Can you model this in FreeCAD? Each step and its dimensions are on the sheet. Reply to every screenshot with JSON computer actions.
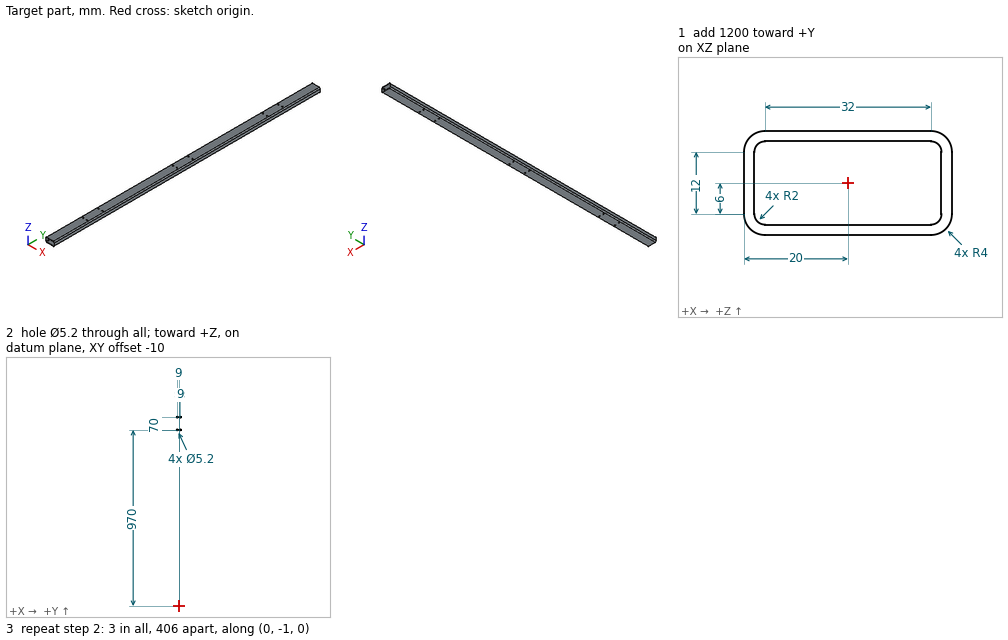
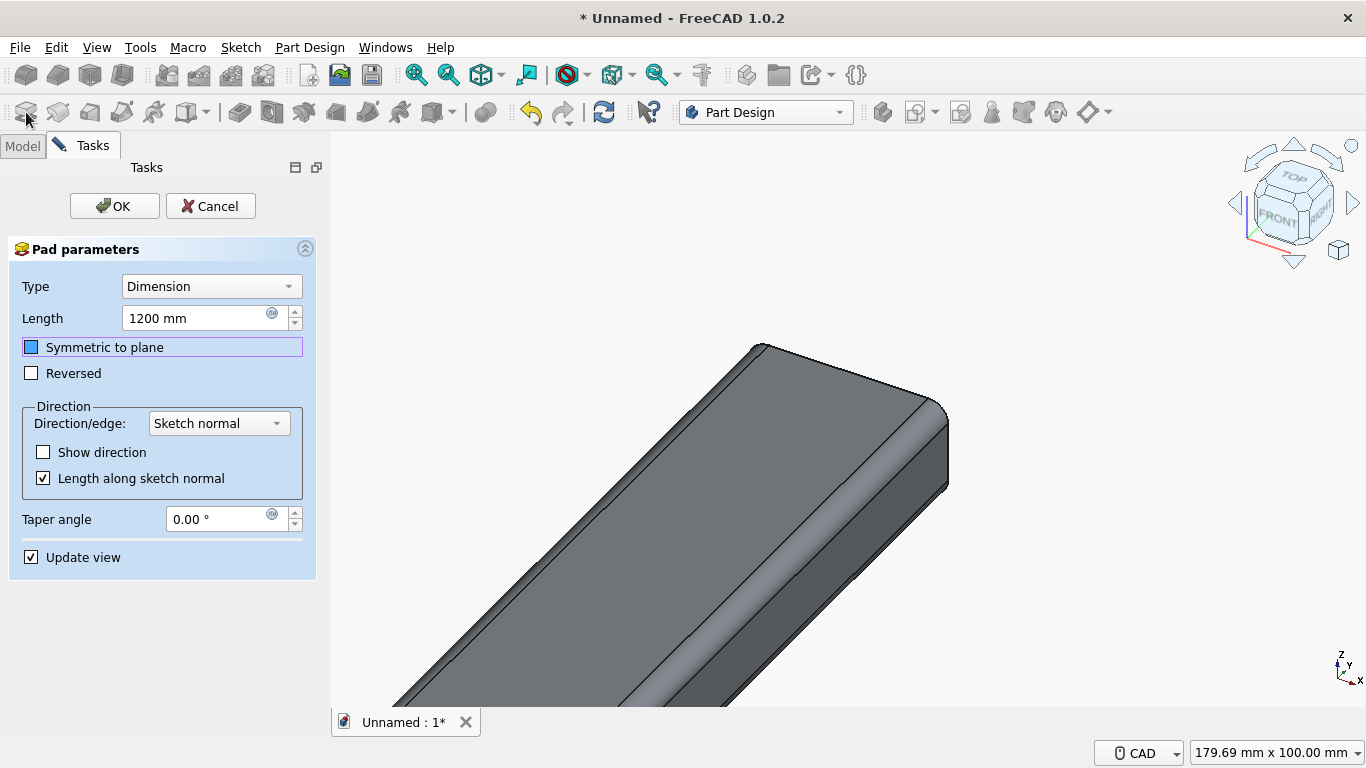
{"action": "left_click", "coordinate": [30, 373]}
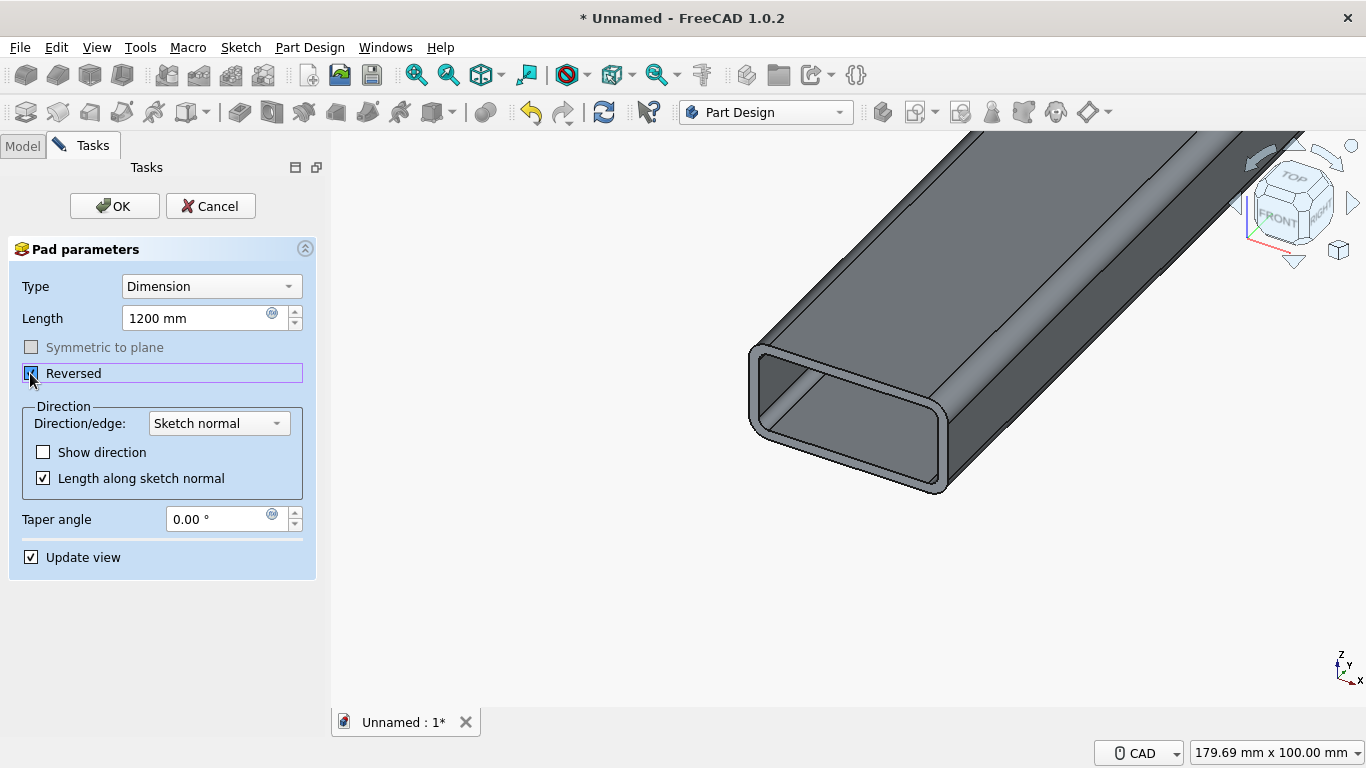
{"action": "left_click", "coordinate": [115, 206]}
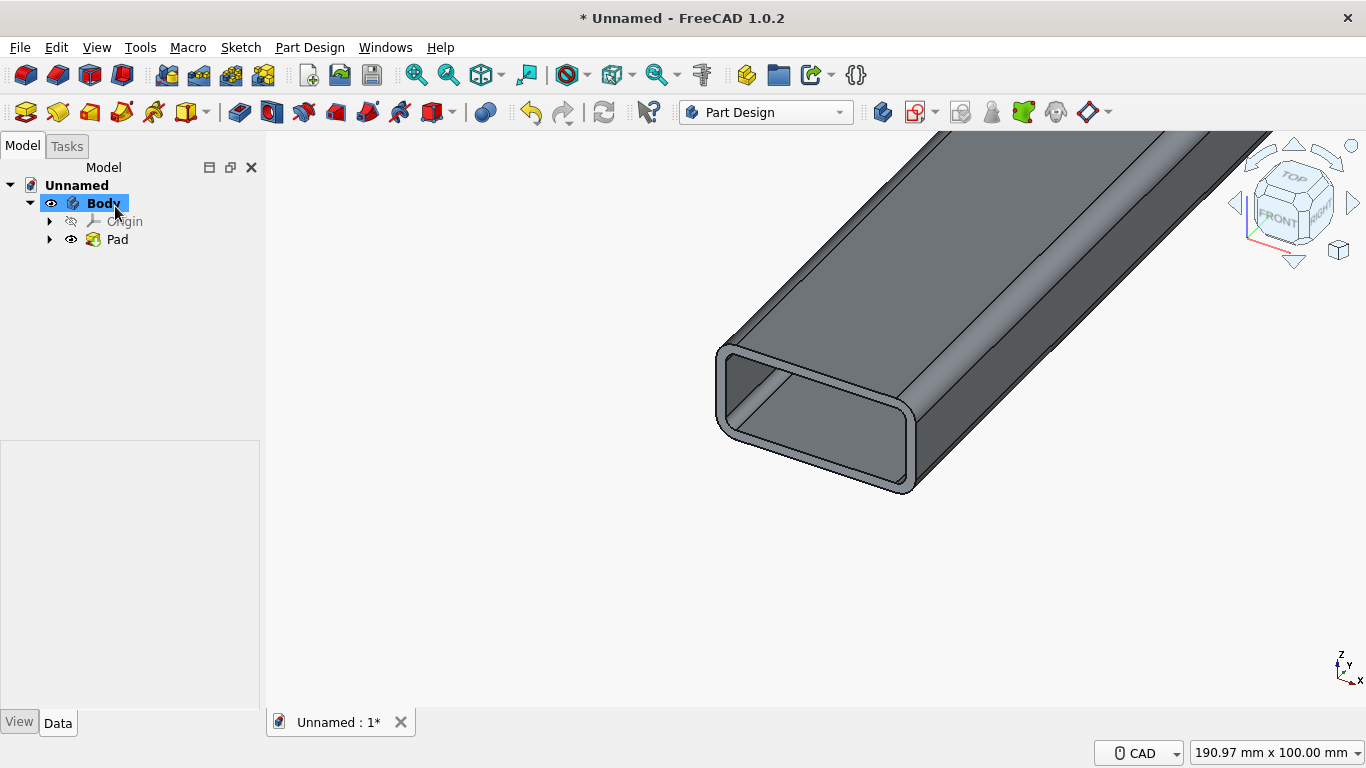
{"action": "key", "text": "v f"}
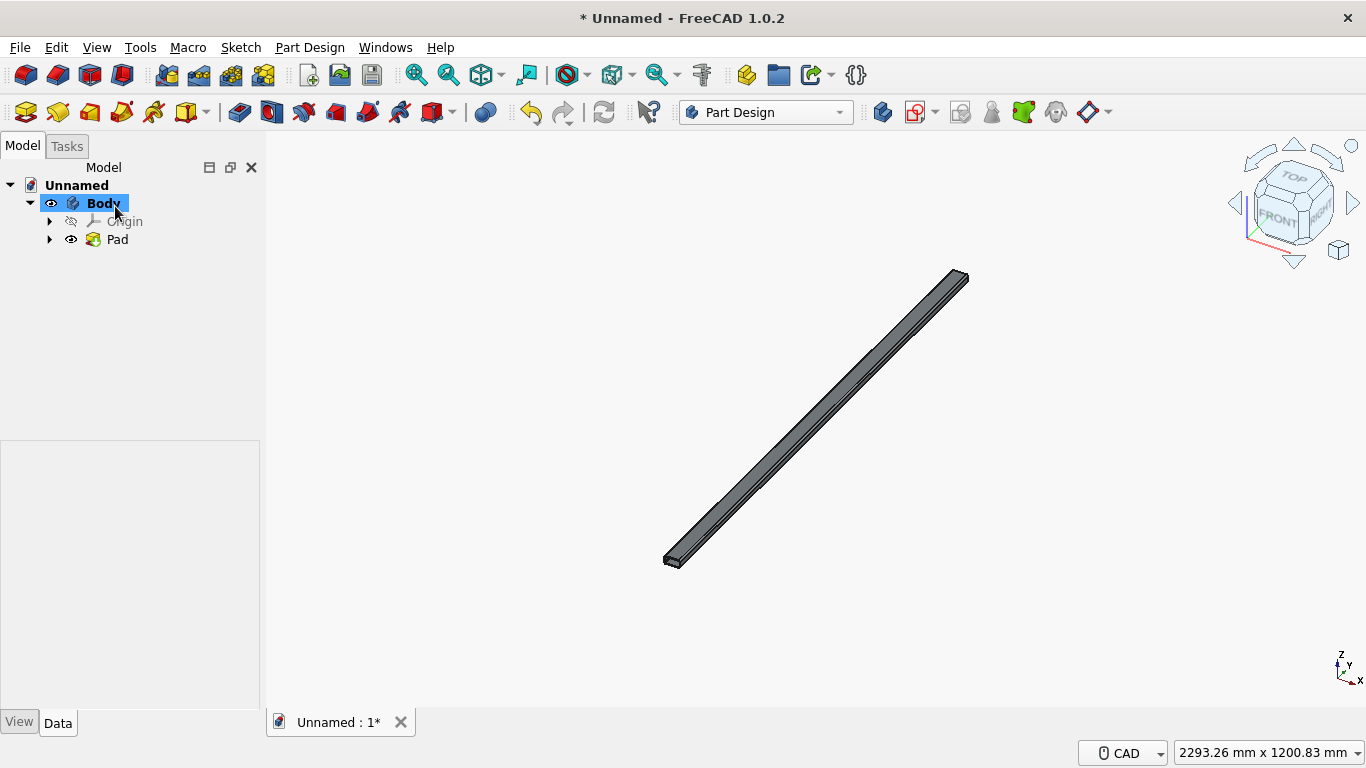
{"action": "key", "text": "5"}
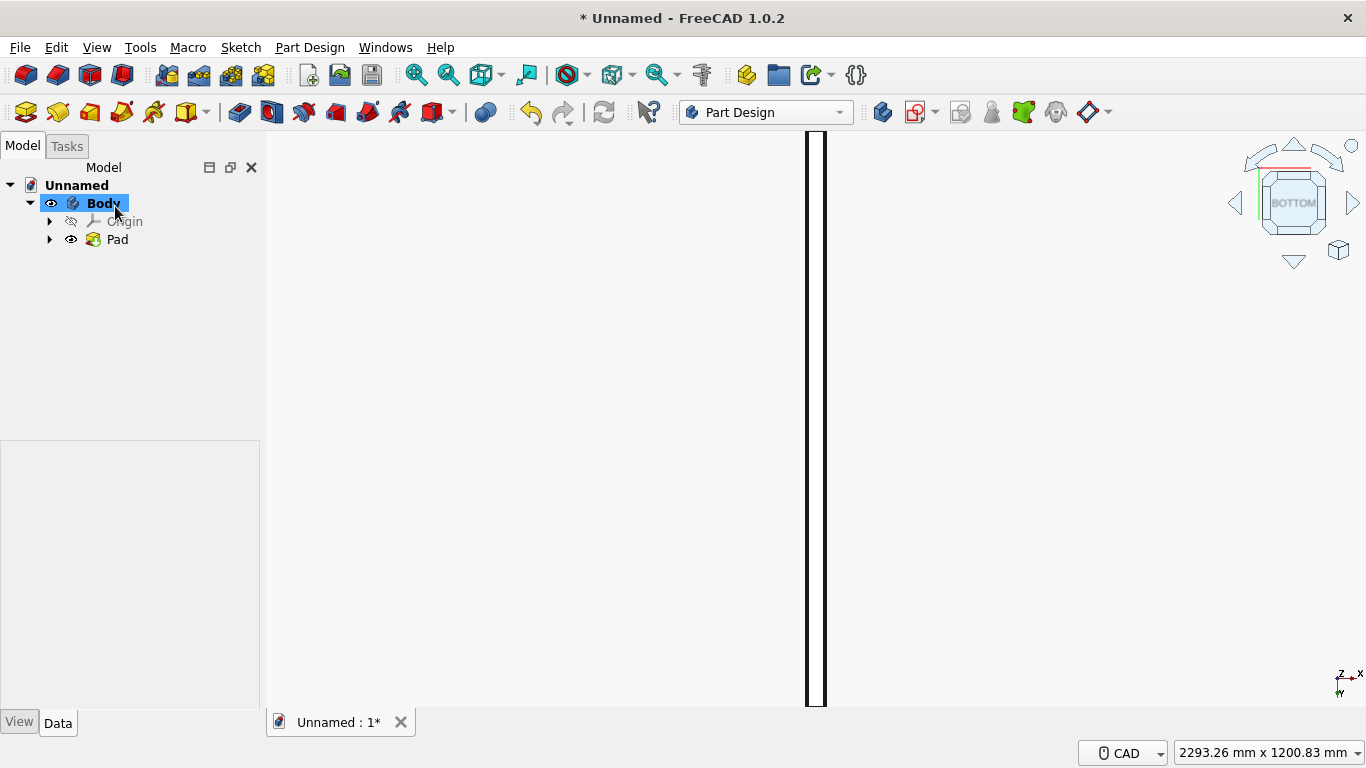
{"action": "left_click", "coordinate": [418, 76]}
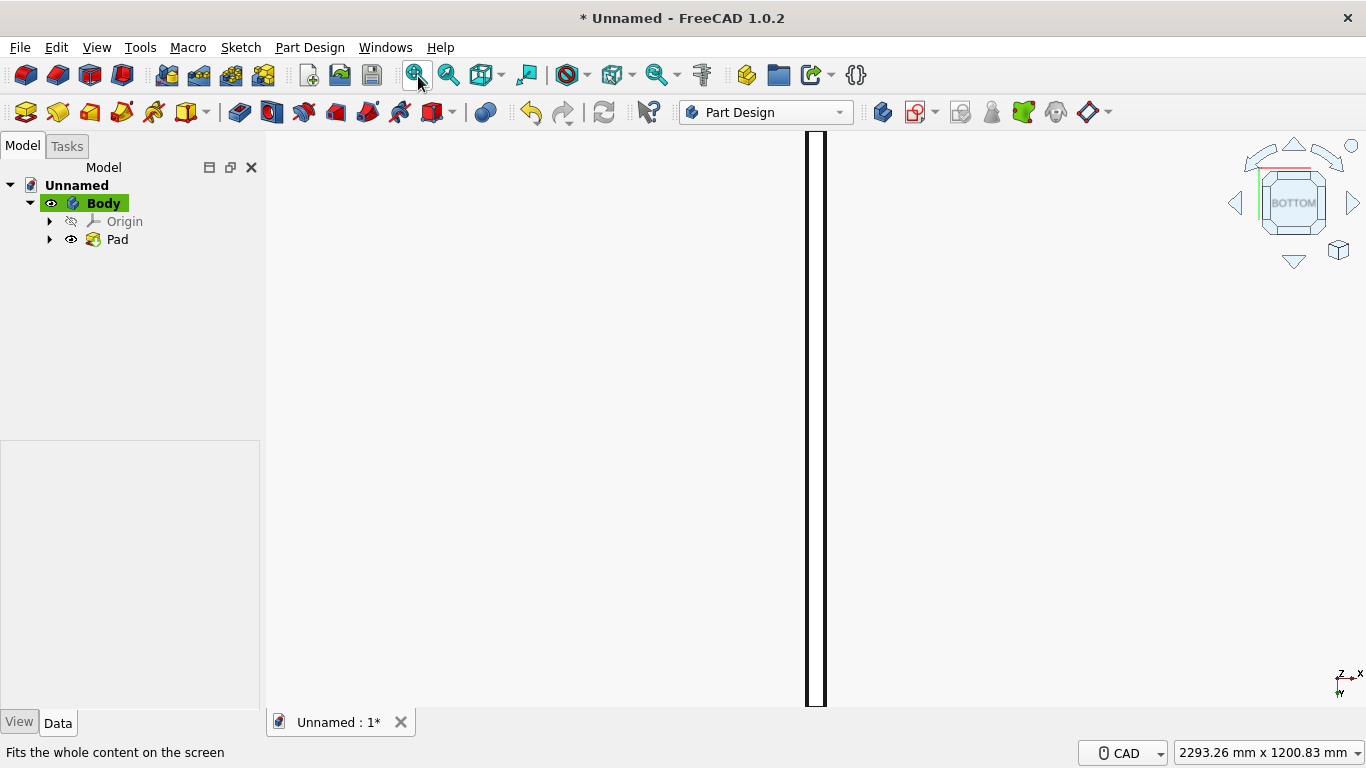
{"action": "key", "text": "1"}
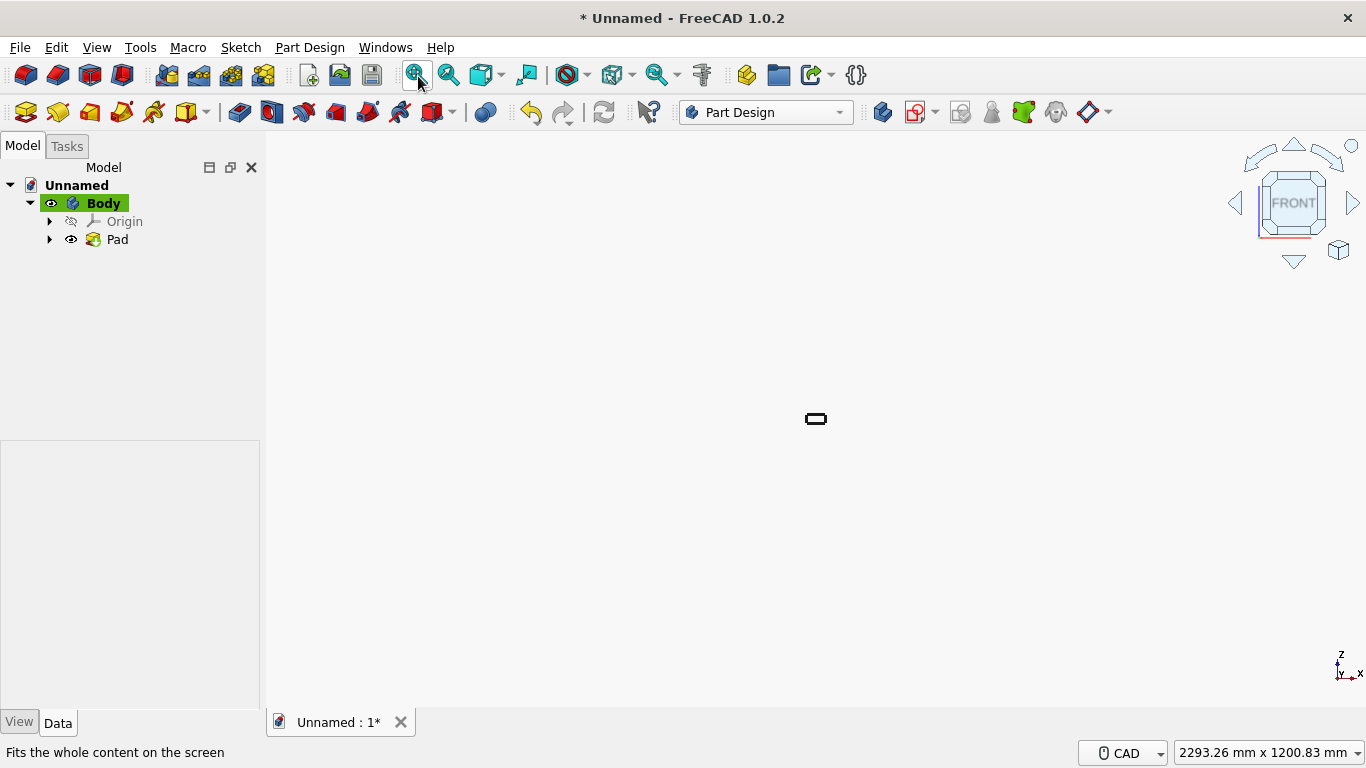
{"action": "left_click", "coordinate": [418, 76]}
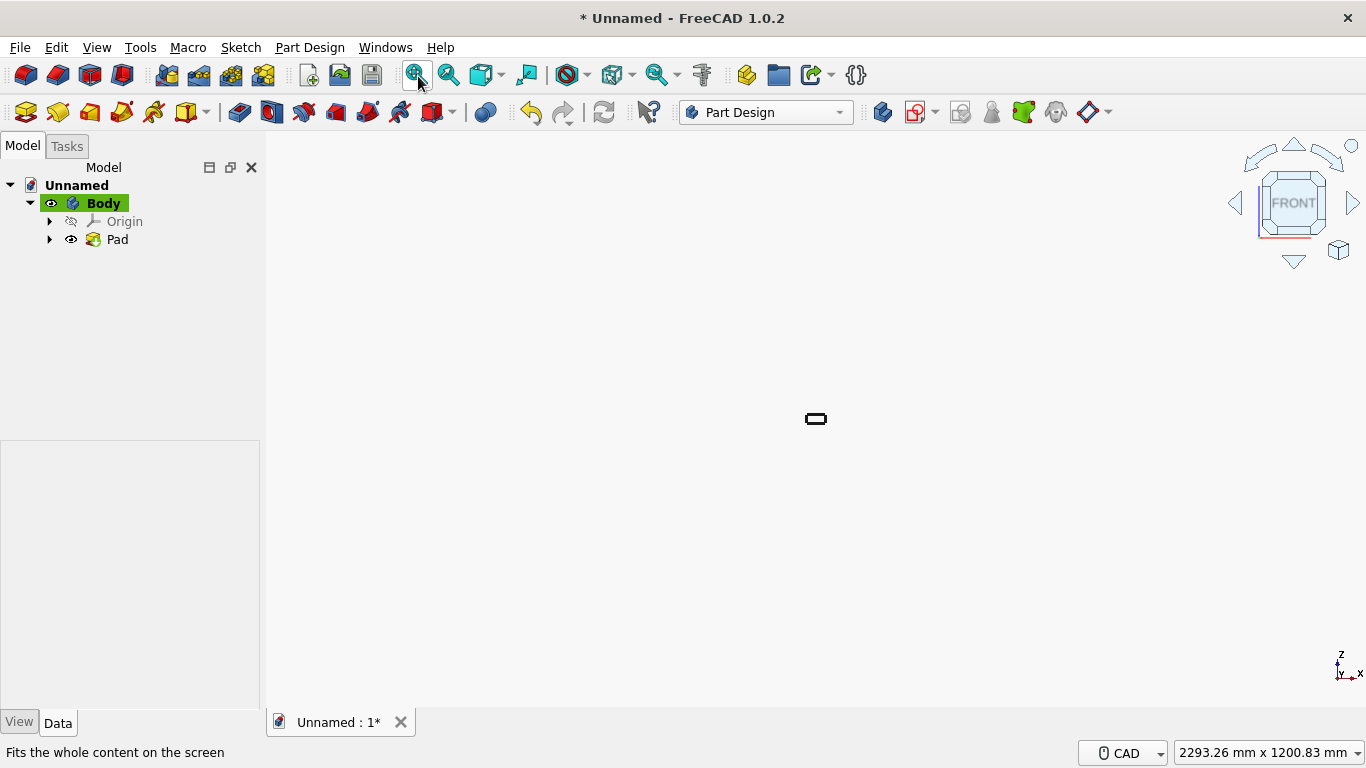
{"action": "key", "text": "3"}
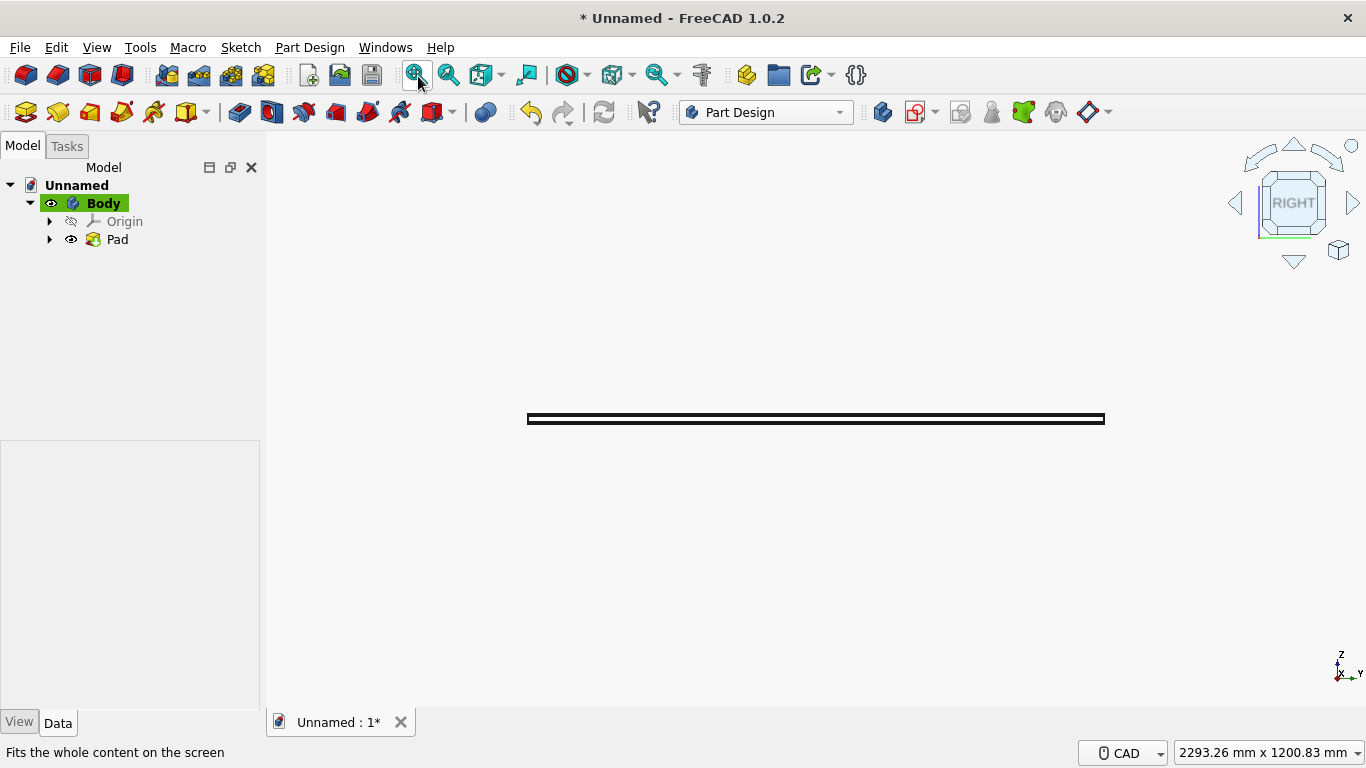
{"action": "left_click", "coordinate": [50, 221]}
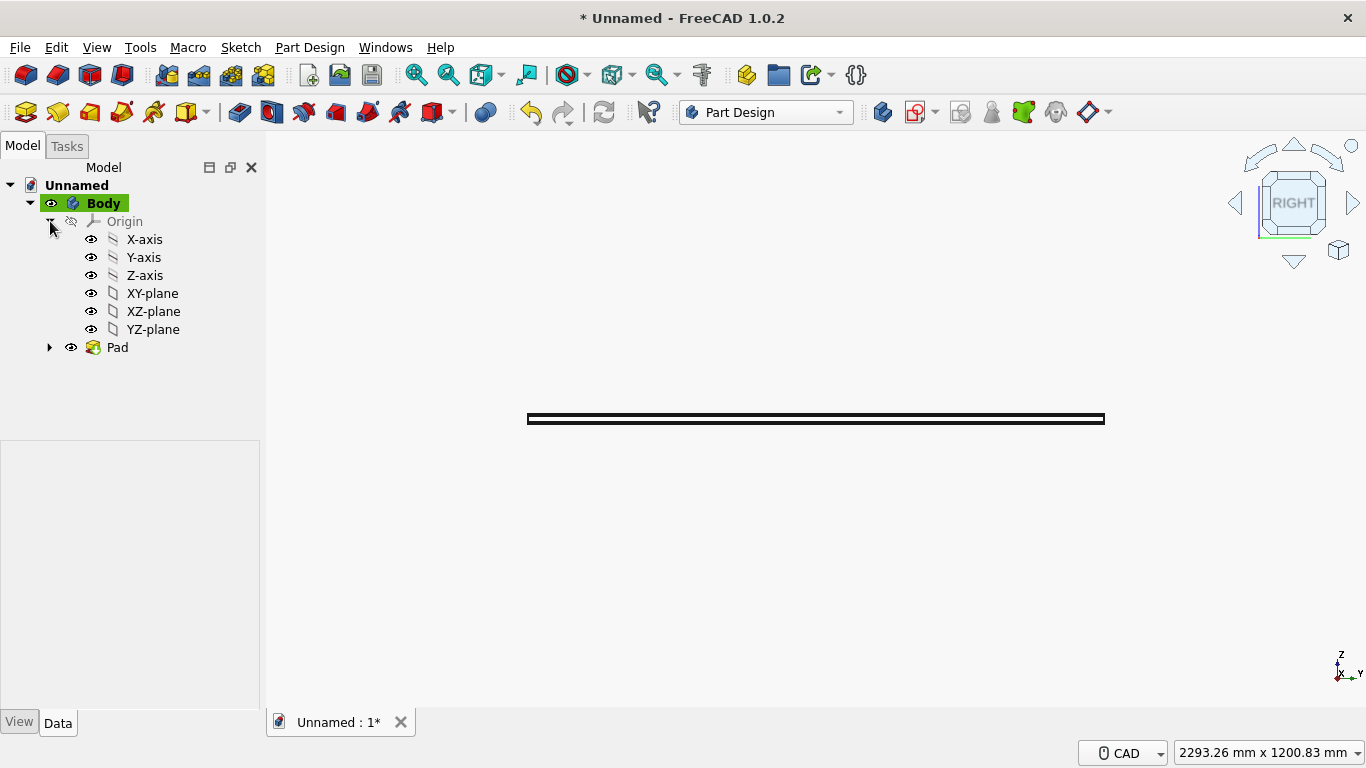
{"action": "left_click", "coordinate": [136, 293]}